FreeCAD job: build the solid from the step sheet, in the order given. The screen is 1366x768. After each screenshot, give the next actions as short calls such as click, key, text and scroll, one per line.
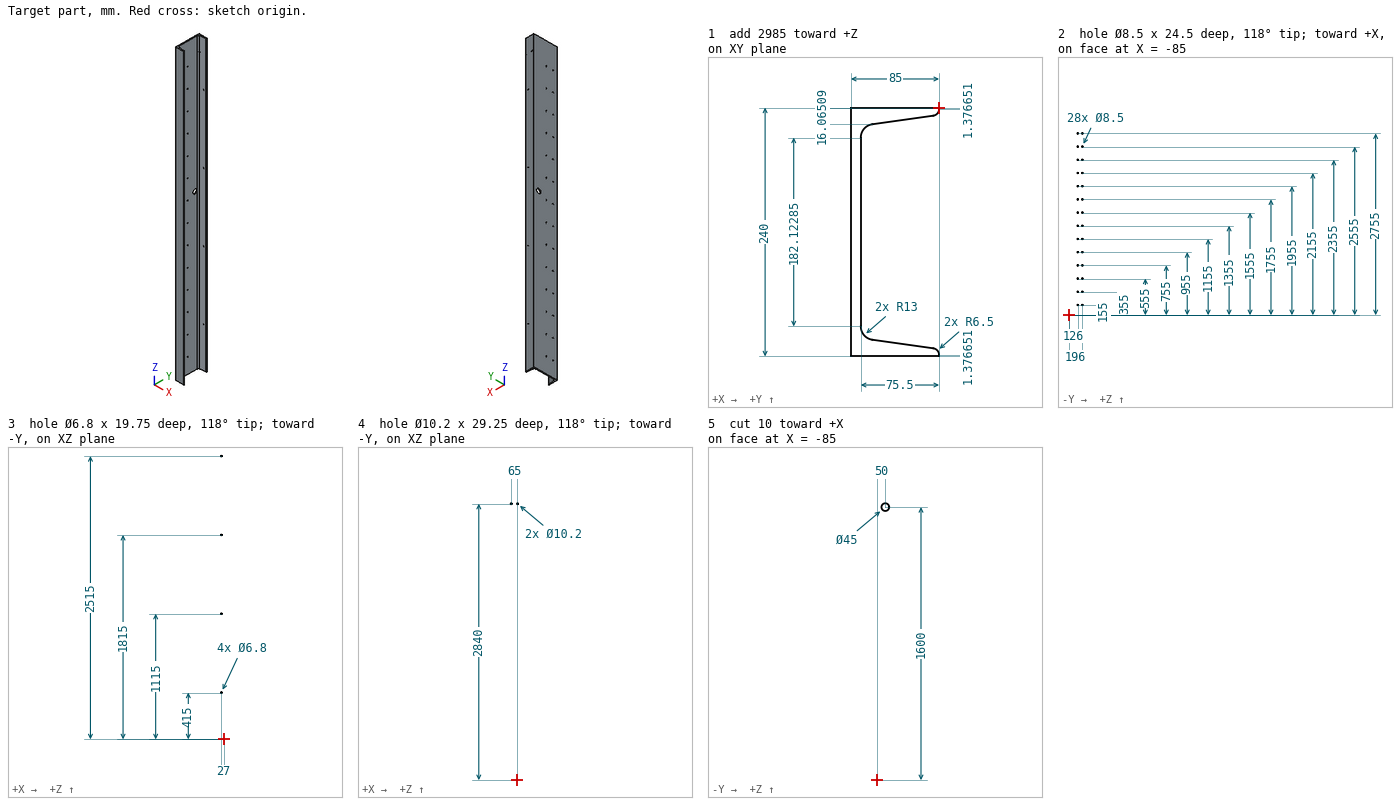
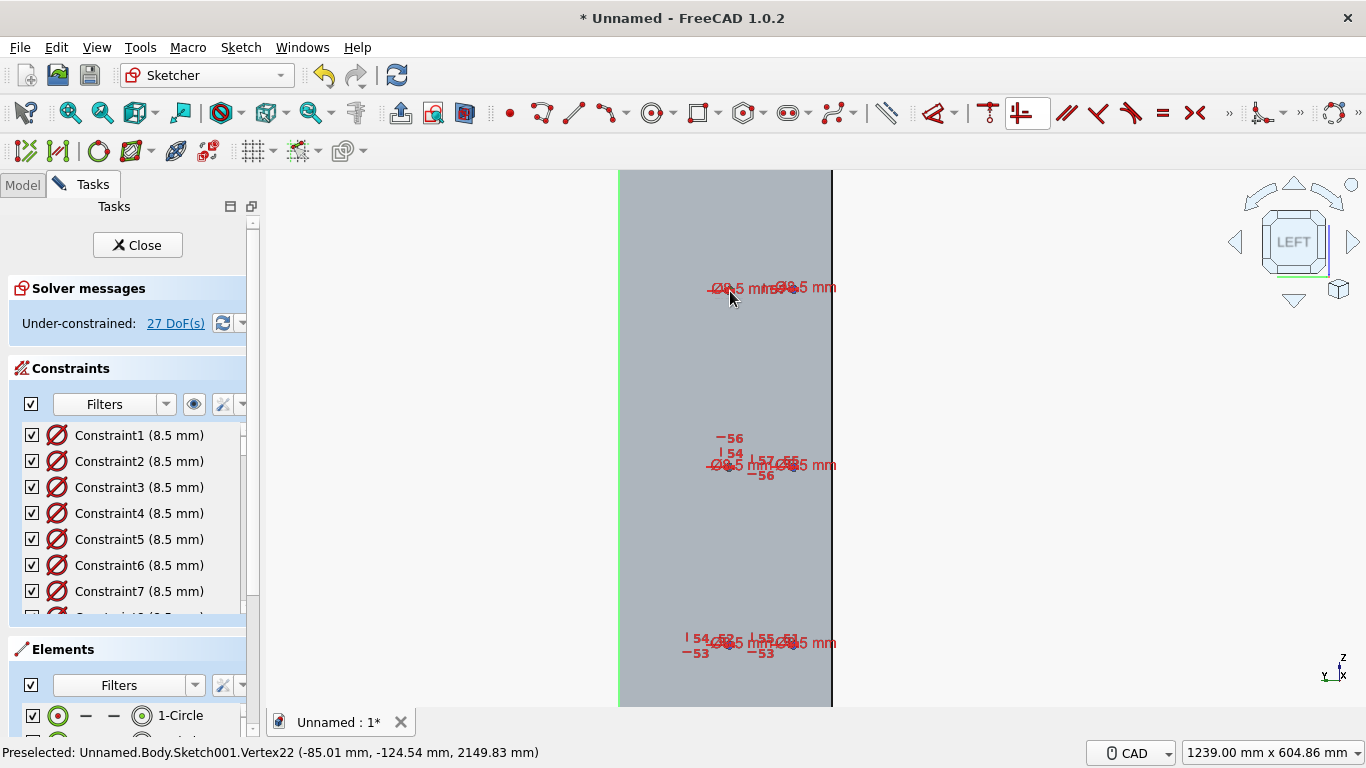
key(v)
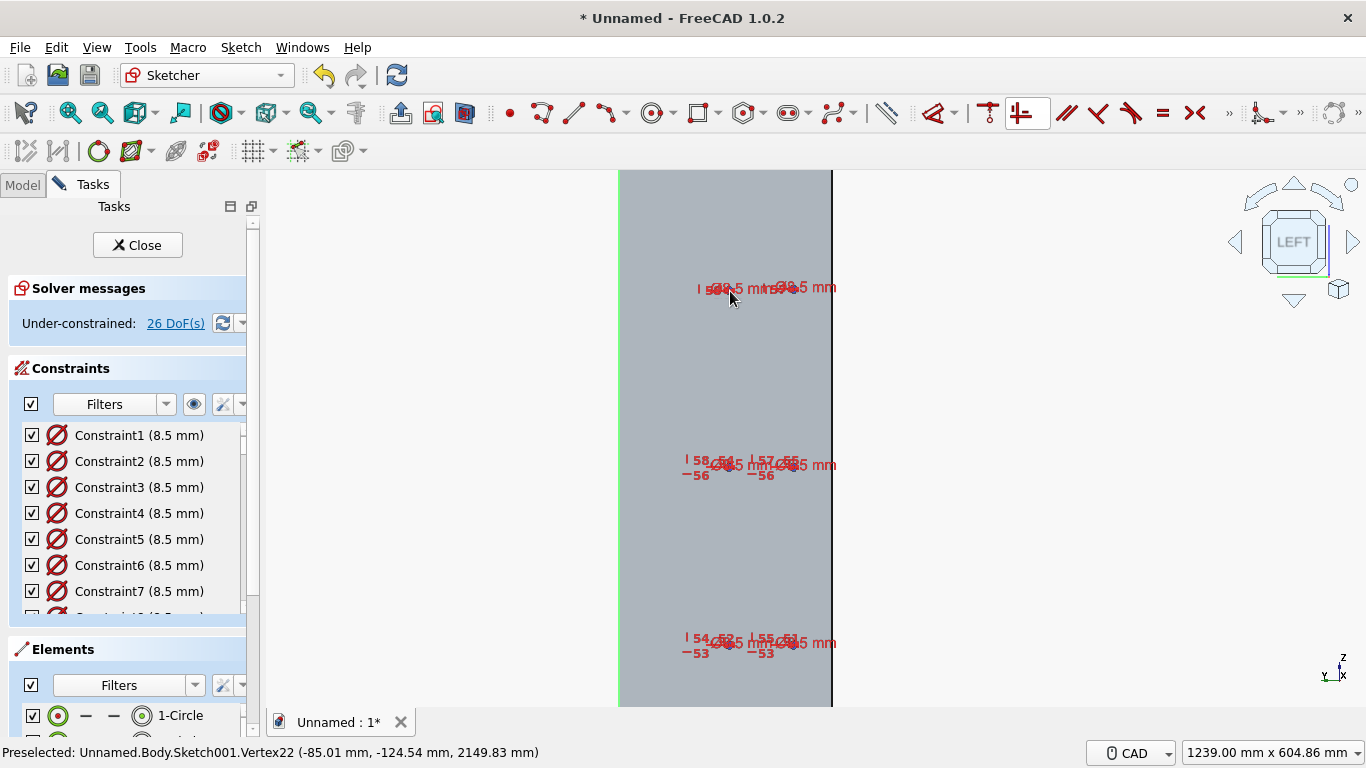
scroll(754, 355, down, 10)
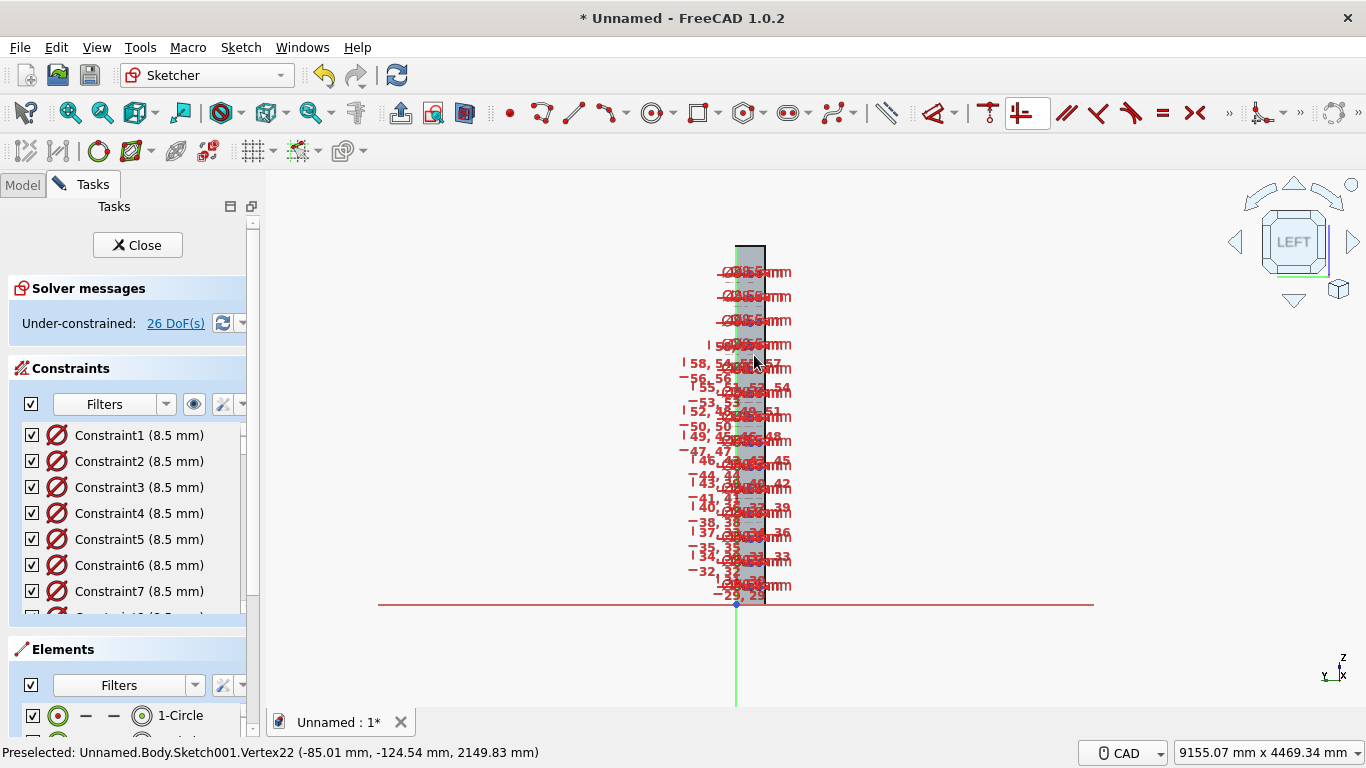
scroll(760, 346, up, 2)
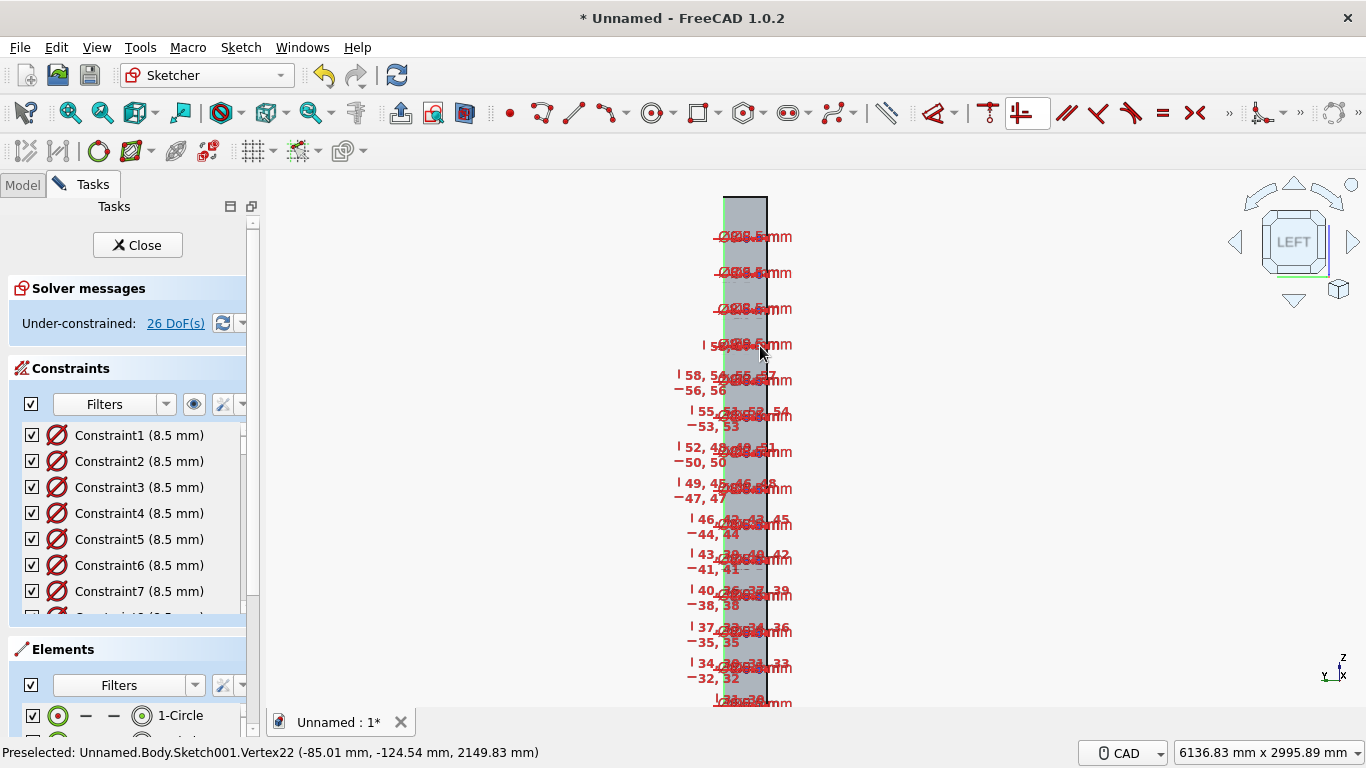
click(759, 346)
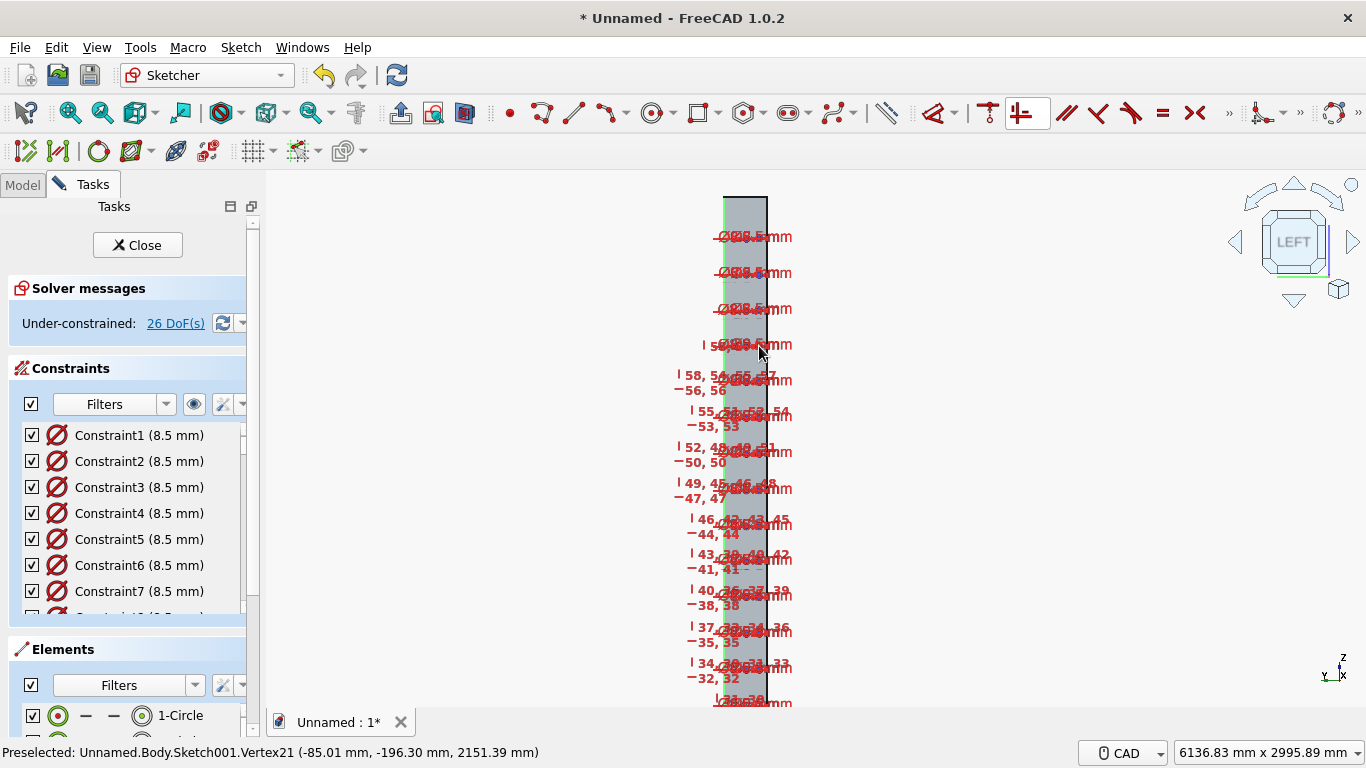
scroll(746, 347, up, 4)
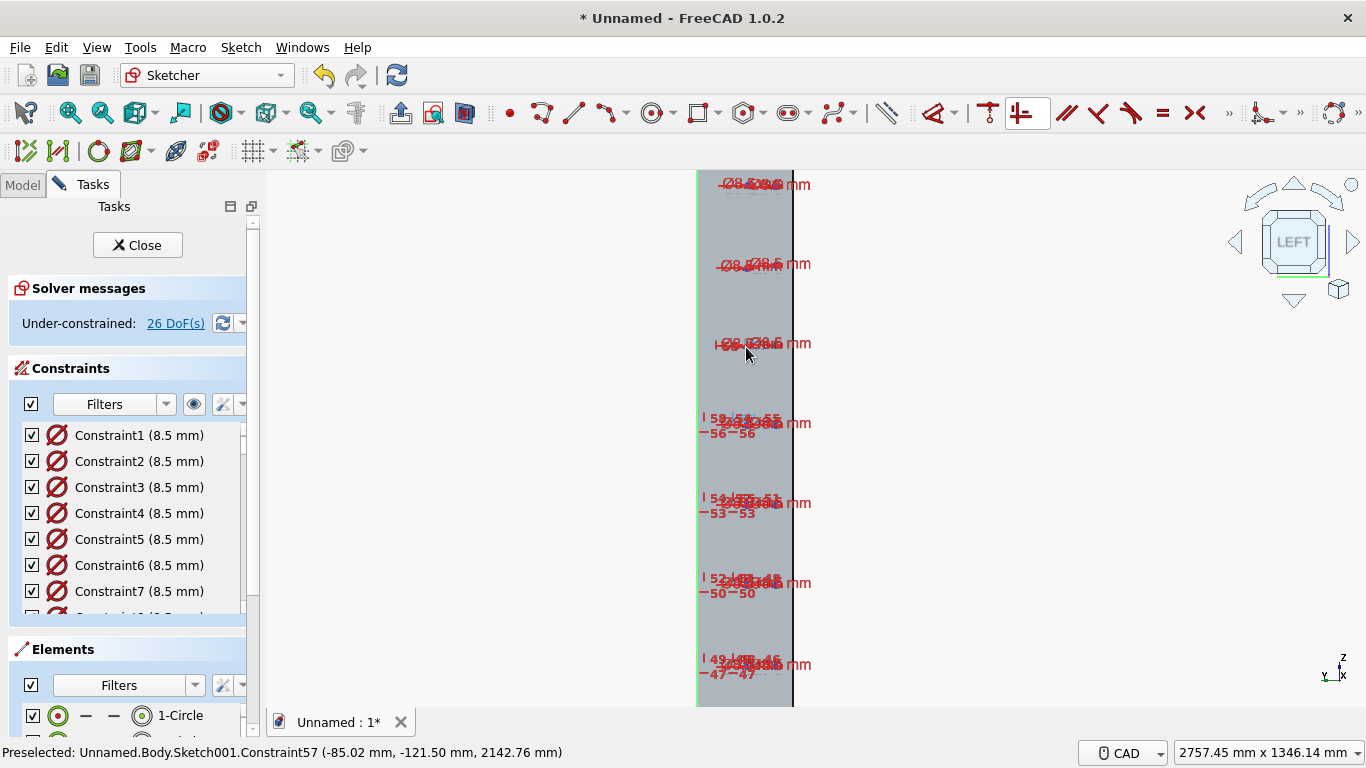
scroll(746, 346, up, 4)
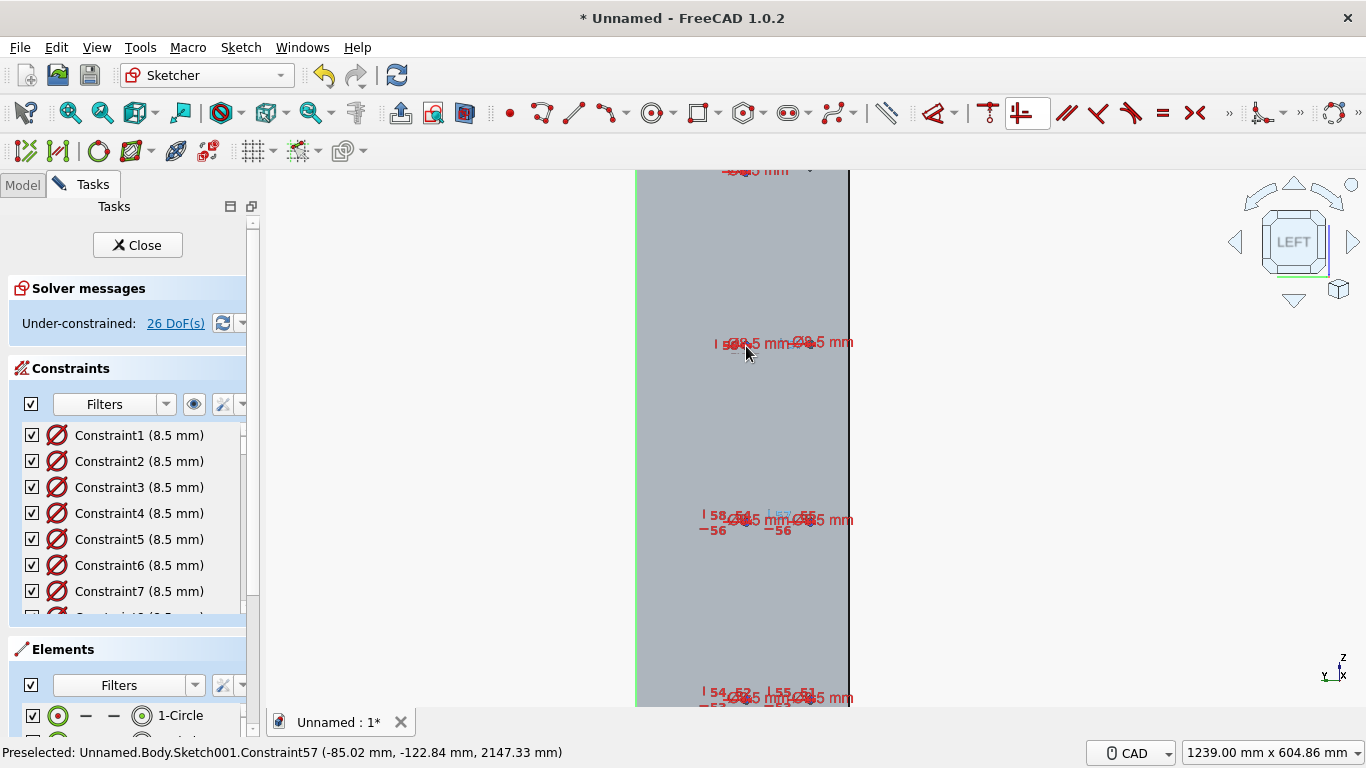
click(746, 346)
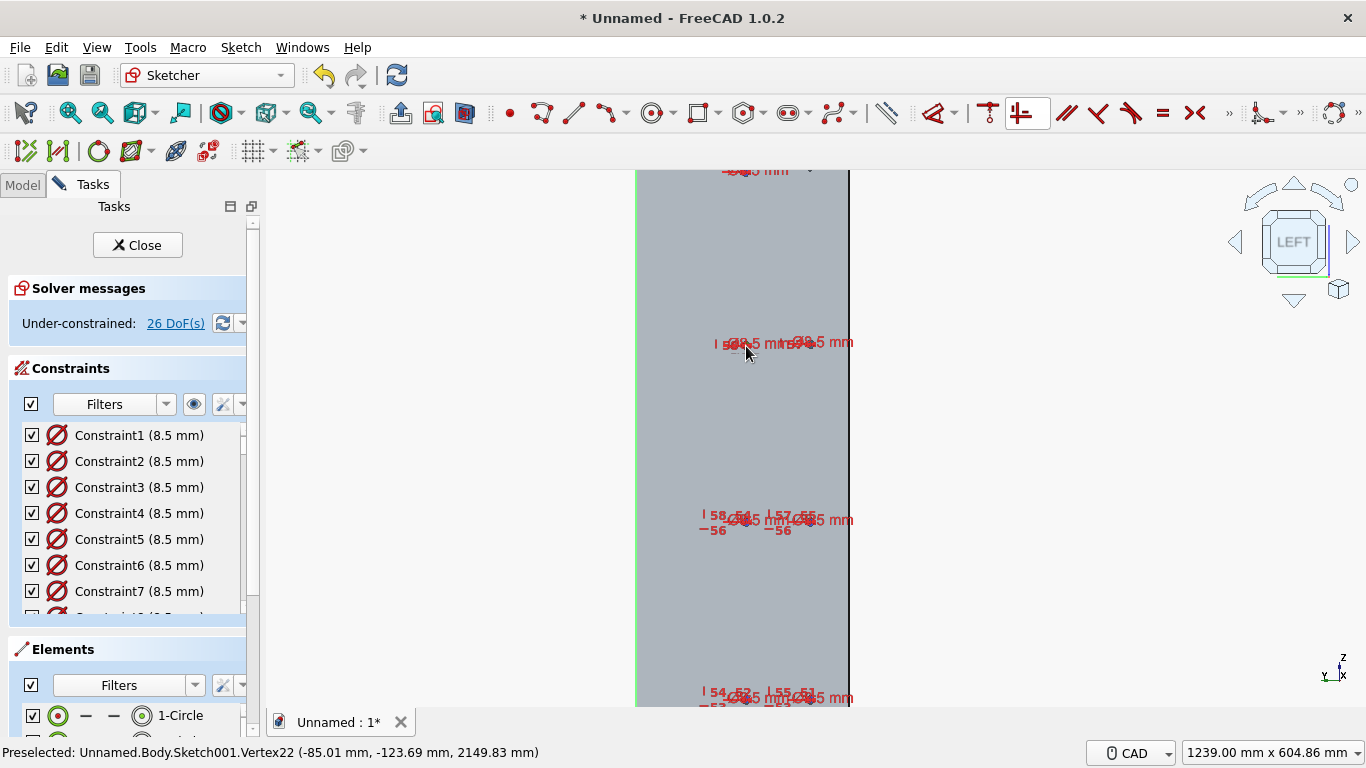
click(1044, 114)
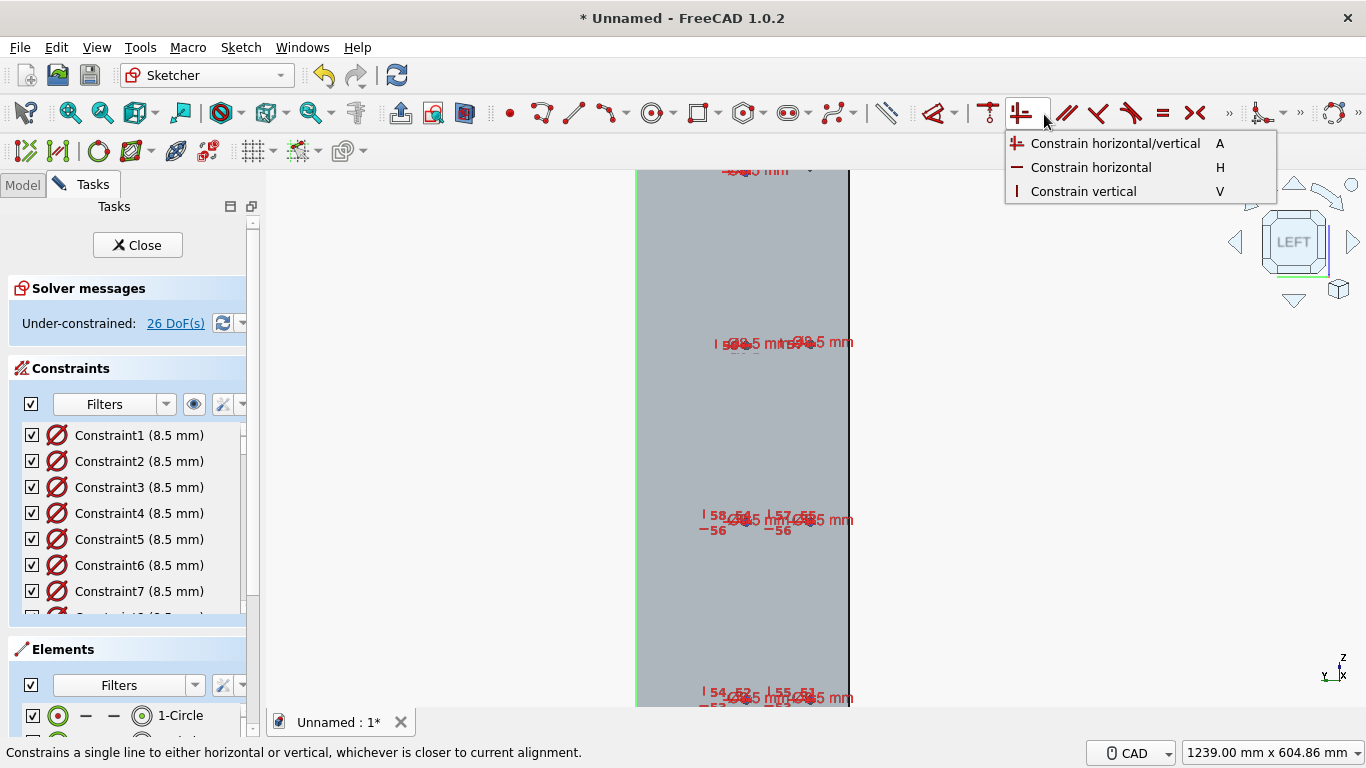
click(1141, 167)